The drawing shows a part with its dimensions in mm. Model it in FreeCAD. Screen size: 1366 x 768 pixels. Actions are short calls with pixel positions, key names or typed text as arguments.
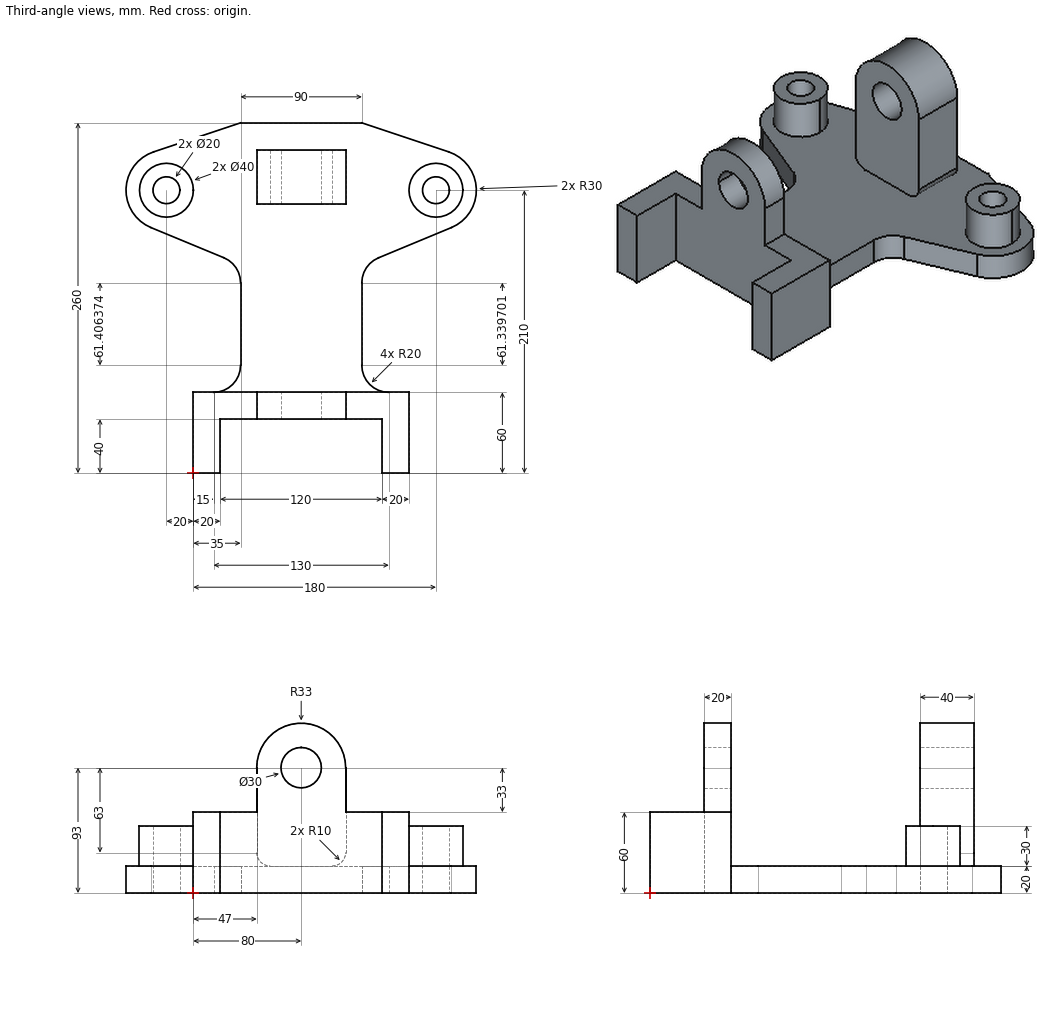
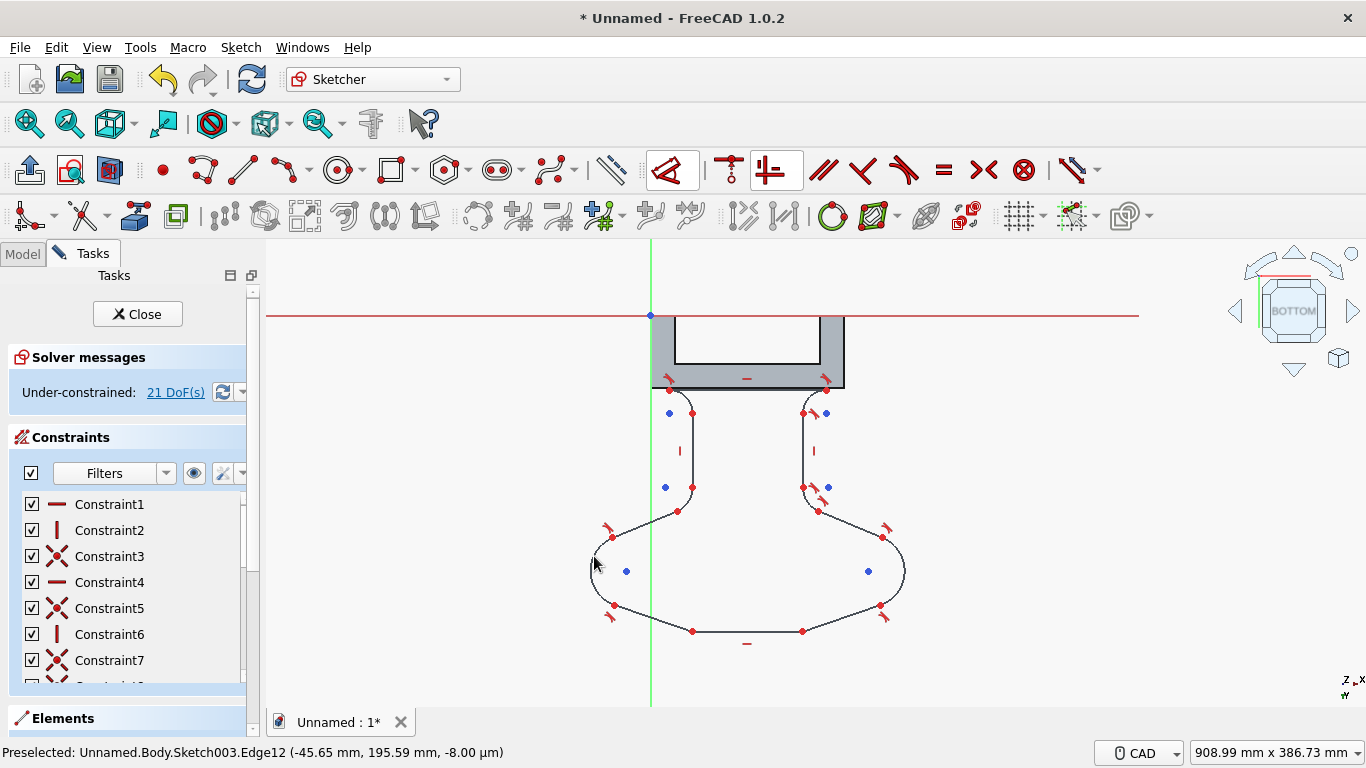
click(632, 530)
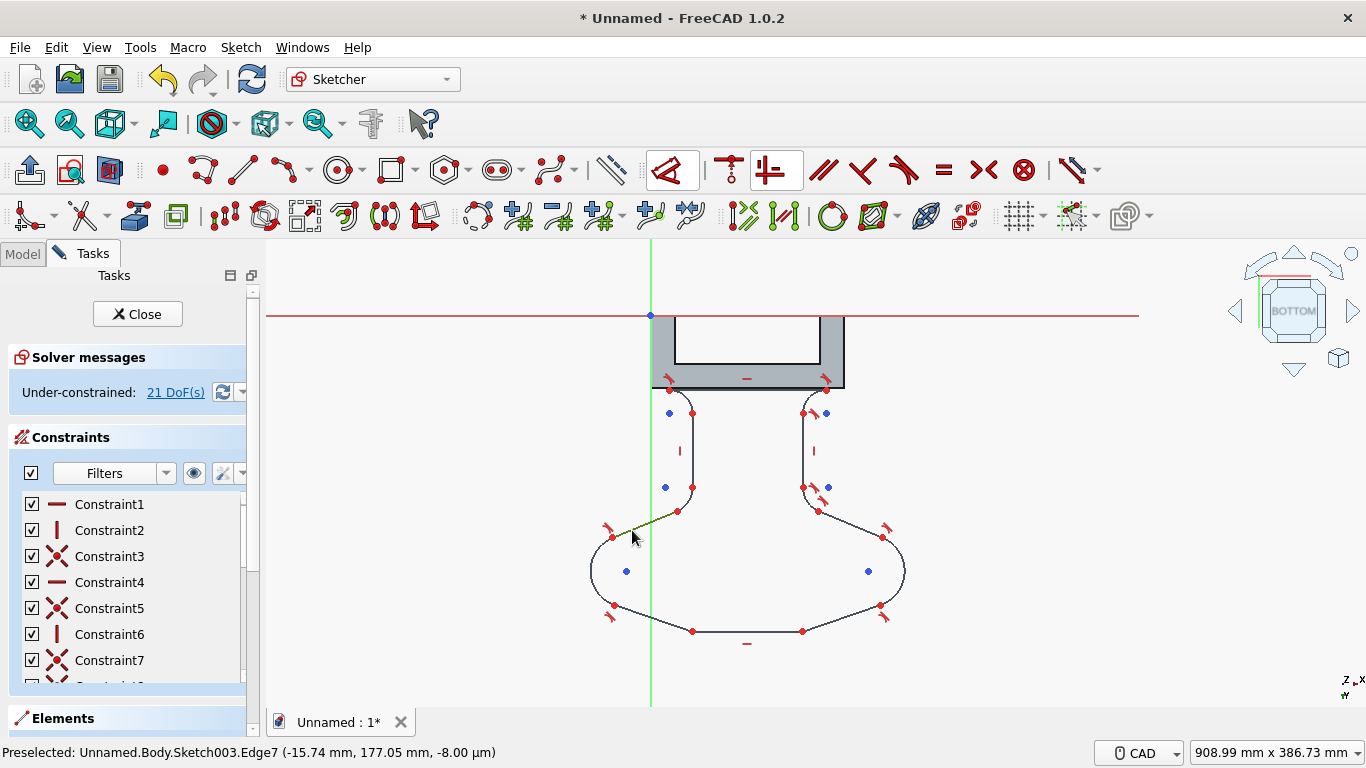
click(688, 501)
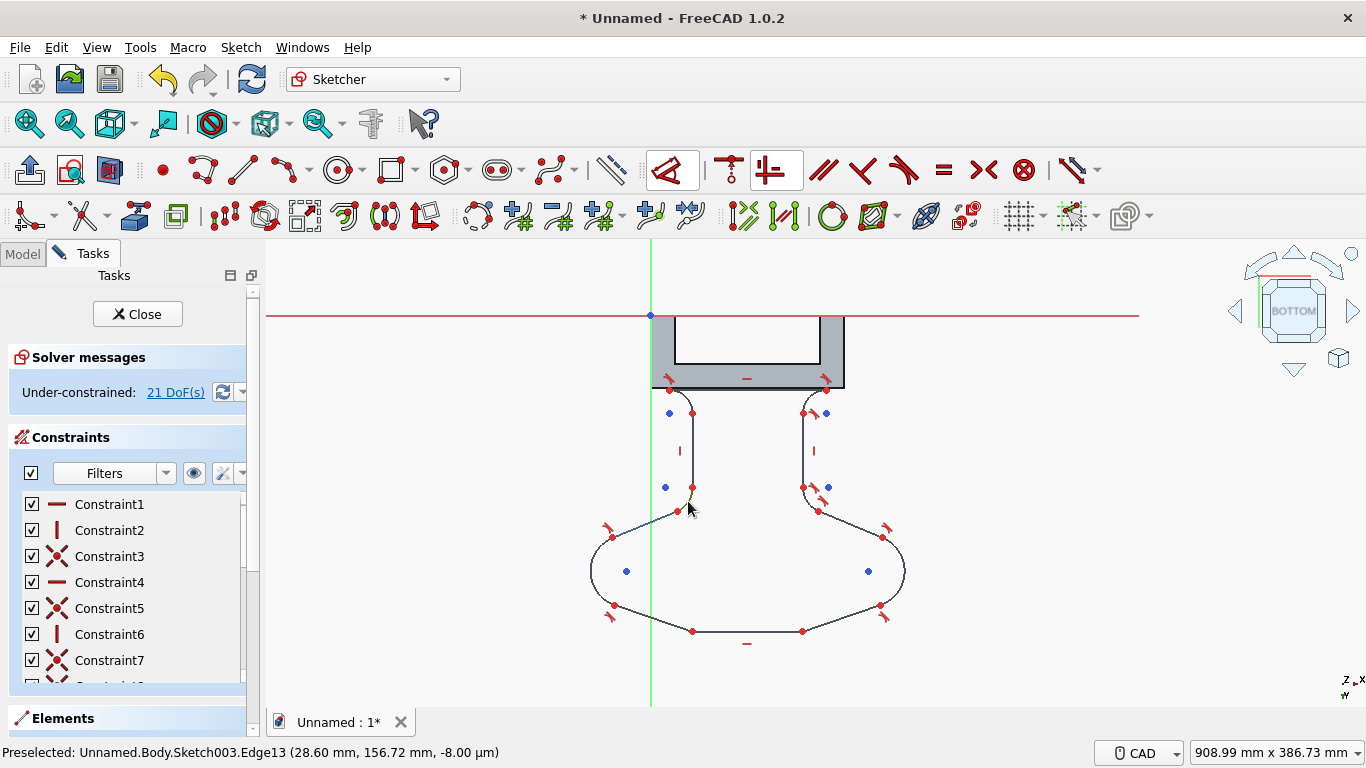
click(904, 170)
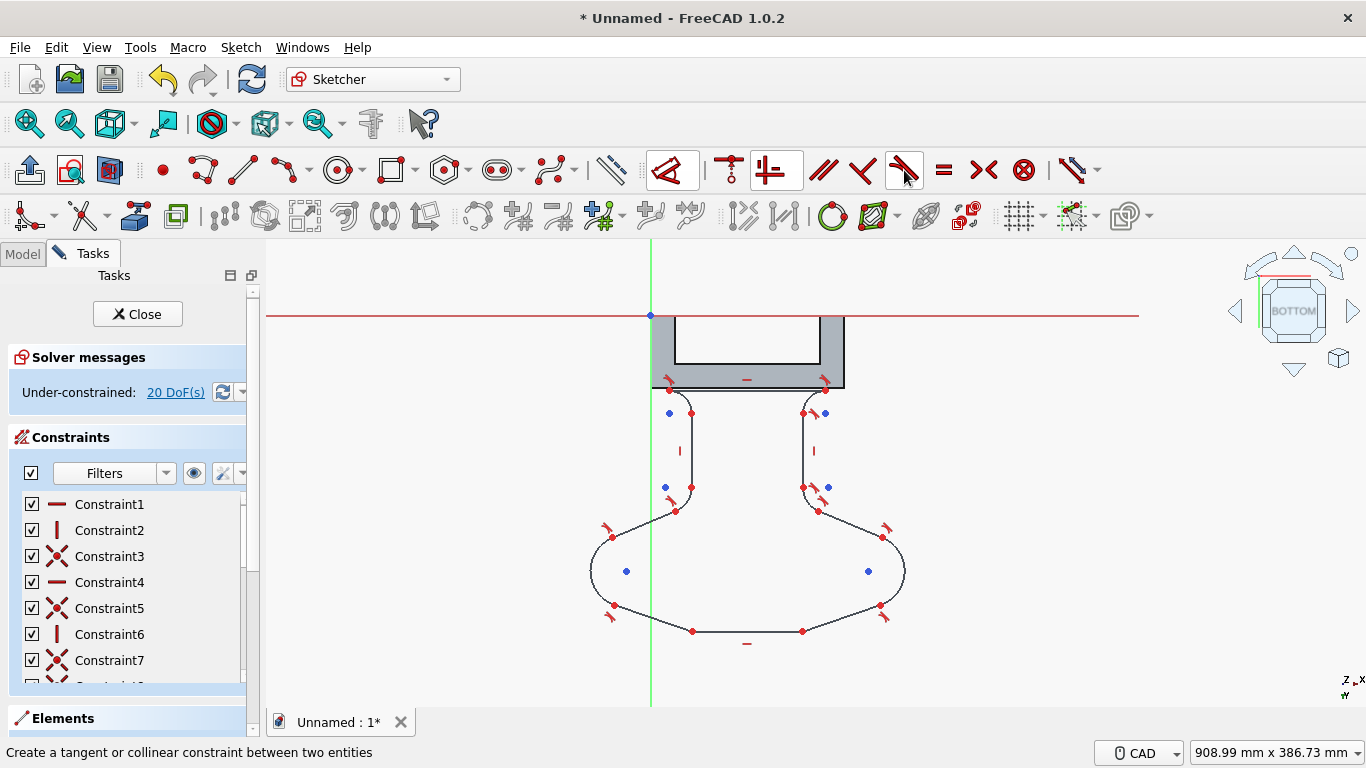
click(692, 465)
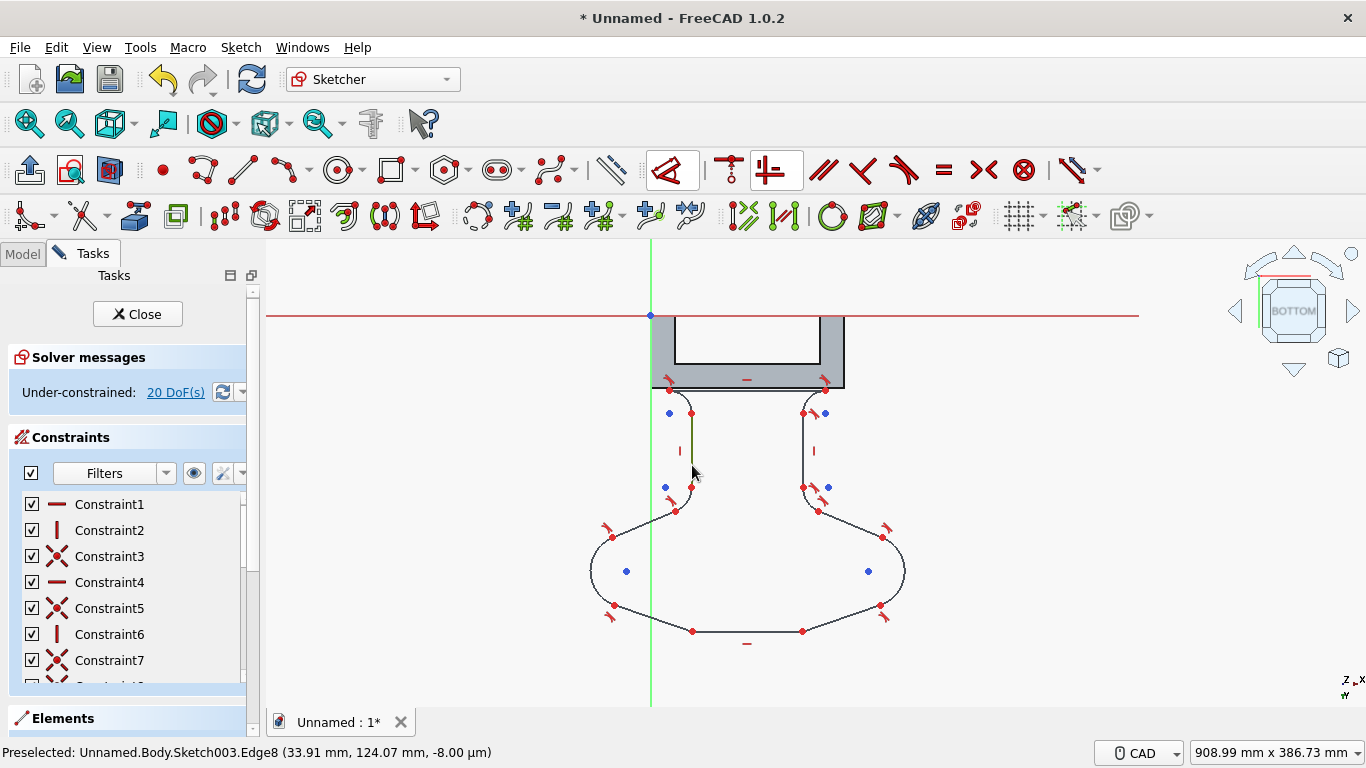
click(687, 502)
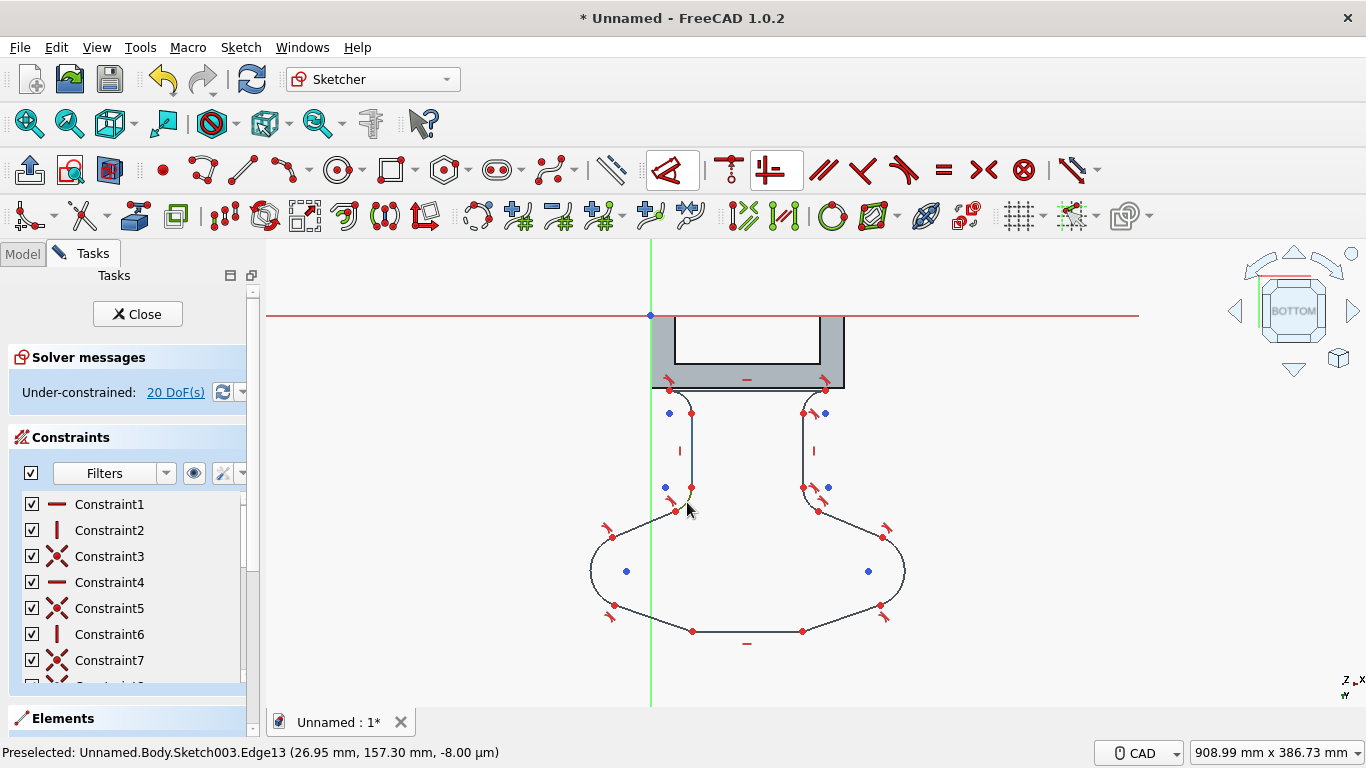
click(904, 170)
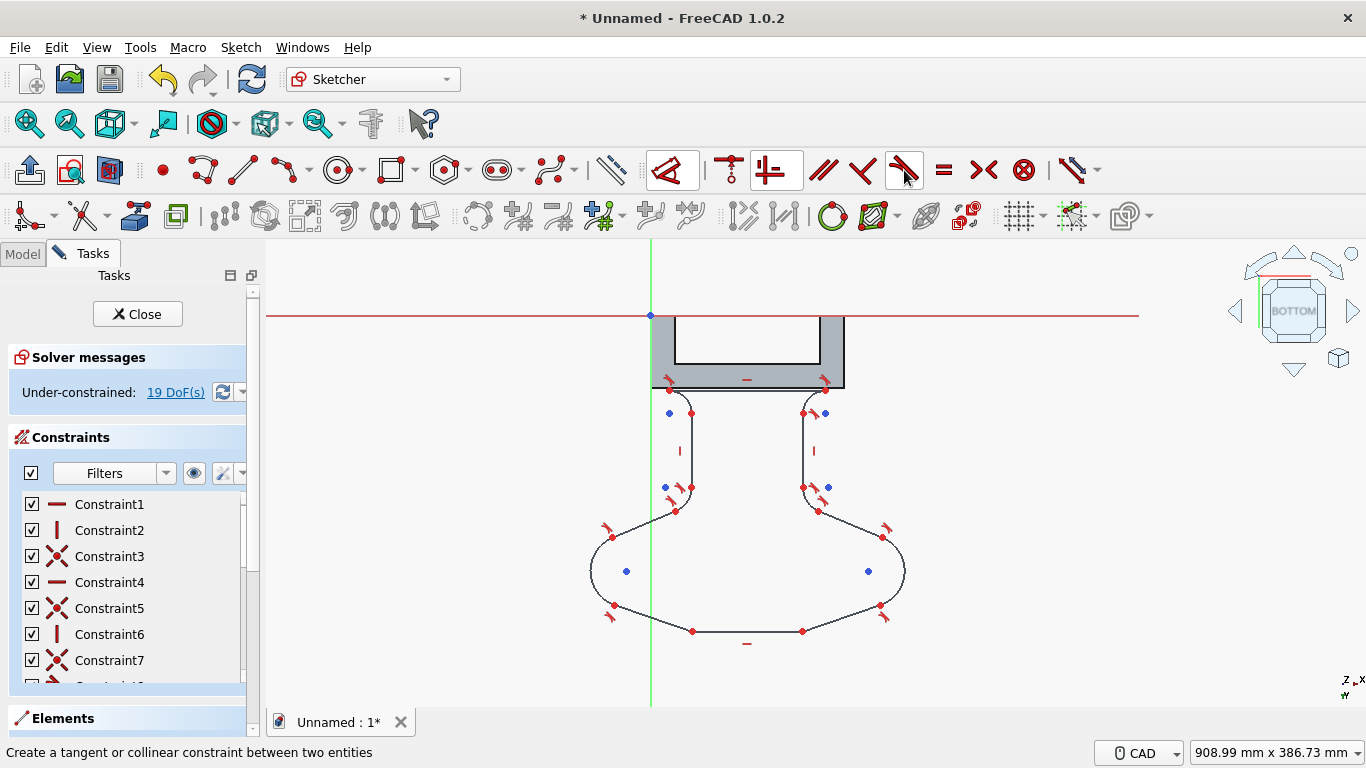
click(692, 465)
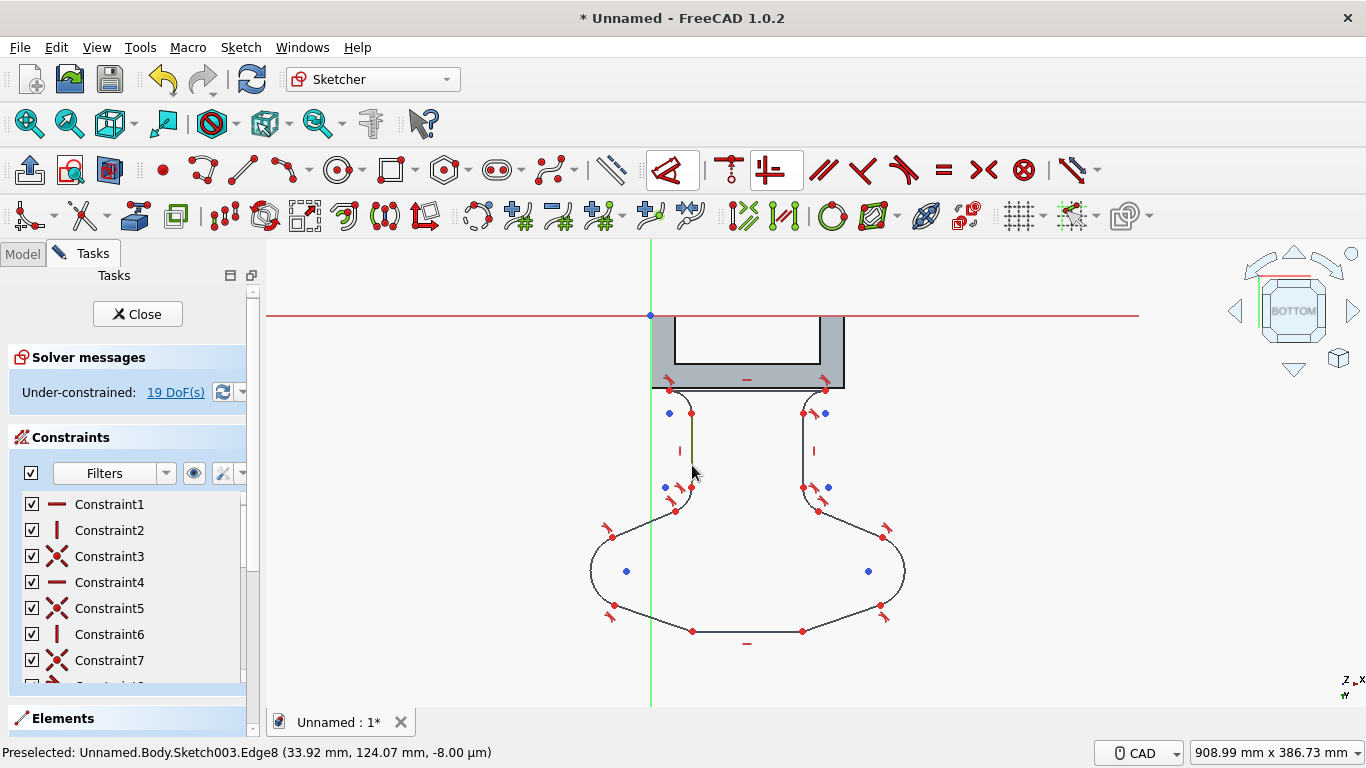
scroll(689, 403, up, 2)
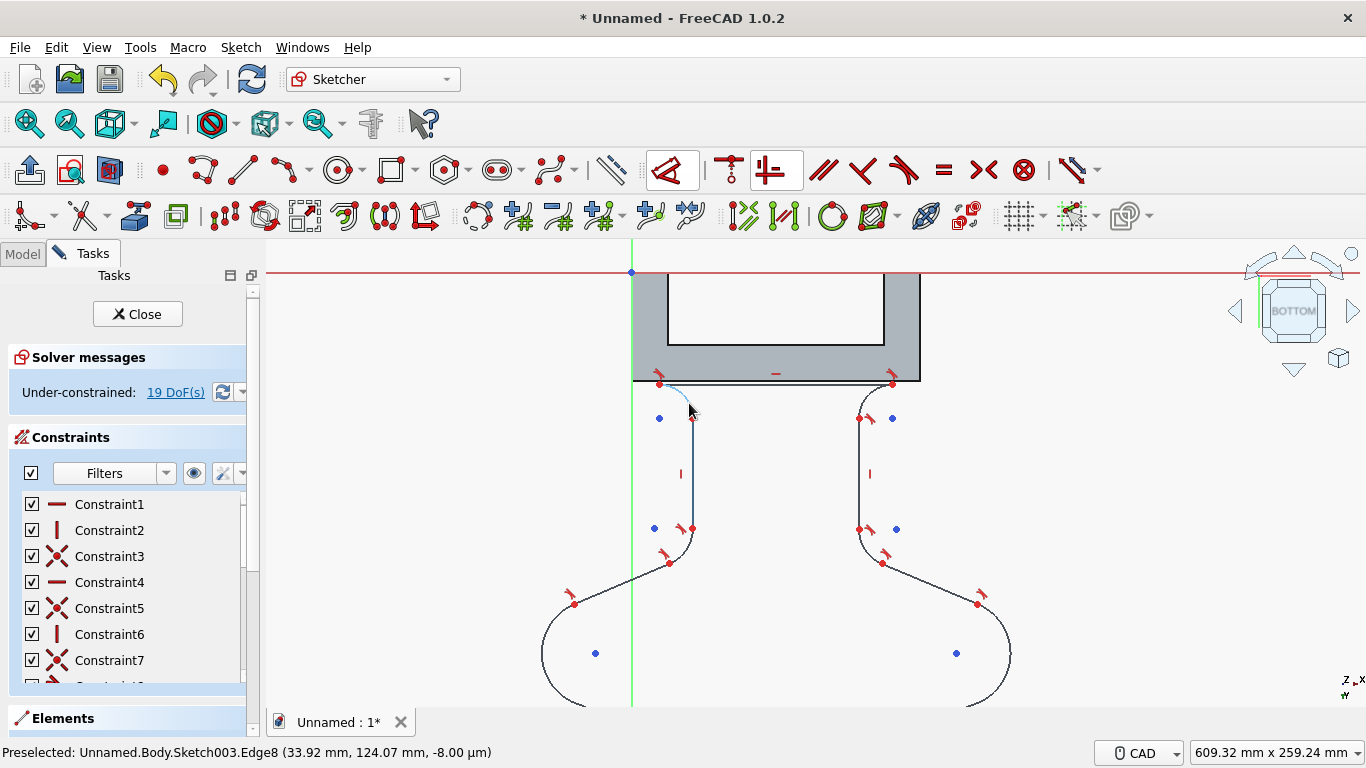
click(689, 403)